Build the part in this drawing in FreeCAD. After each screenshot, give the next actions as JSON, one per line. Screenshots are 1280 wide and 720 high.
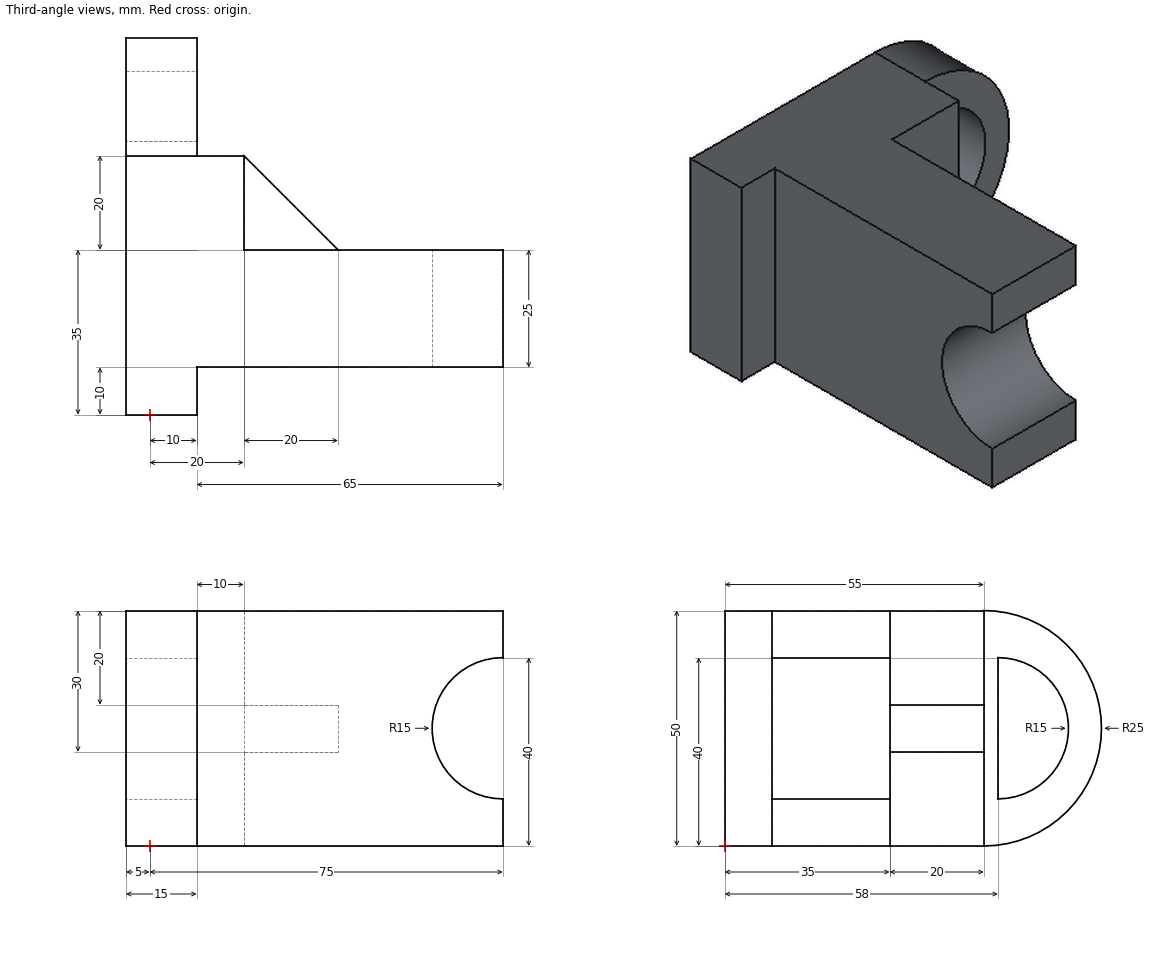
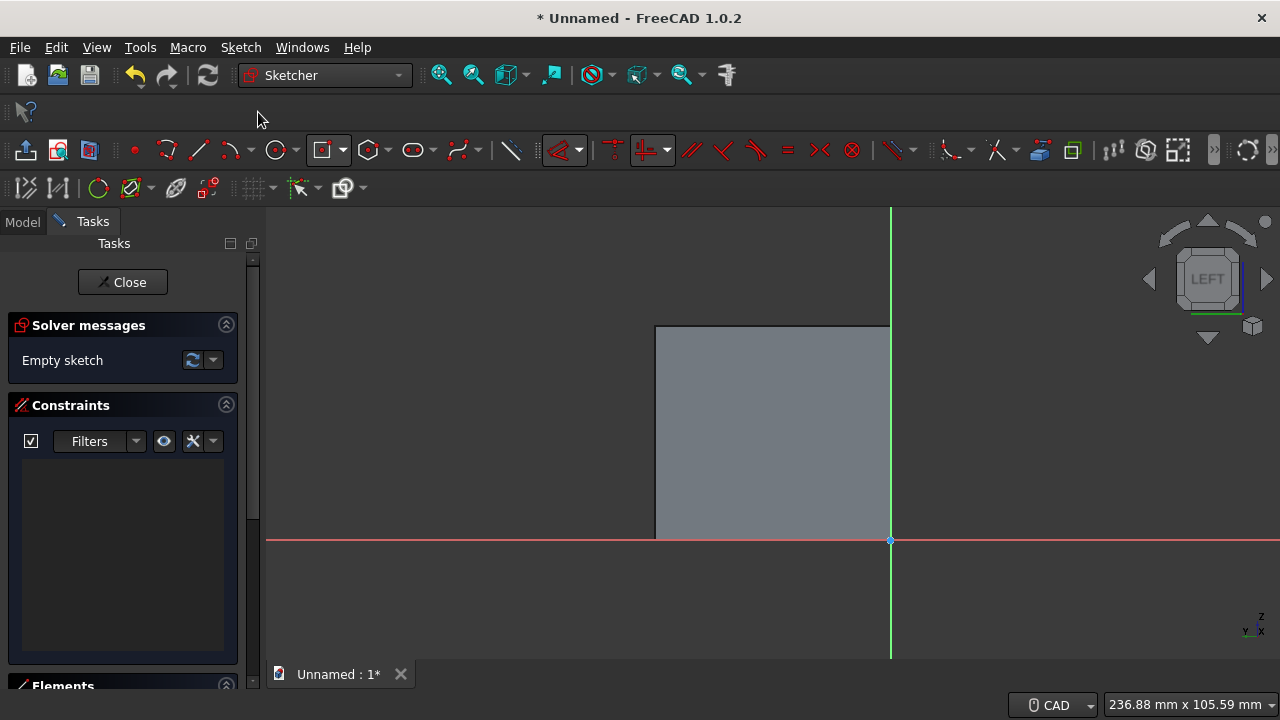
{"action": "left_click", "coordinate": [346, 150]}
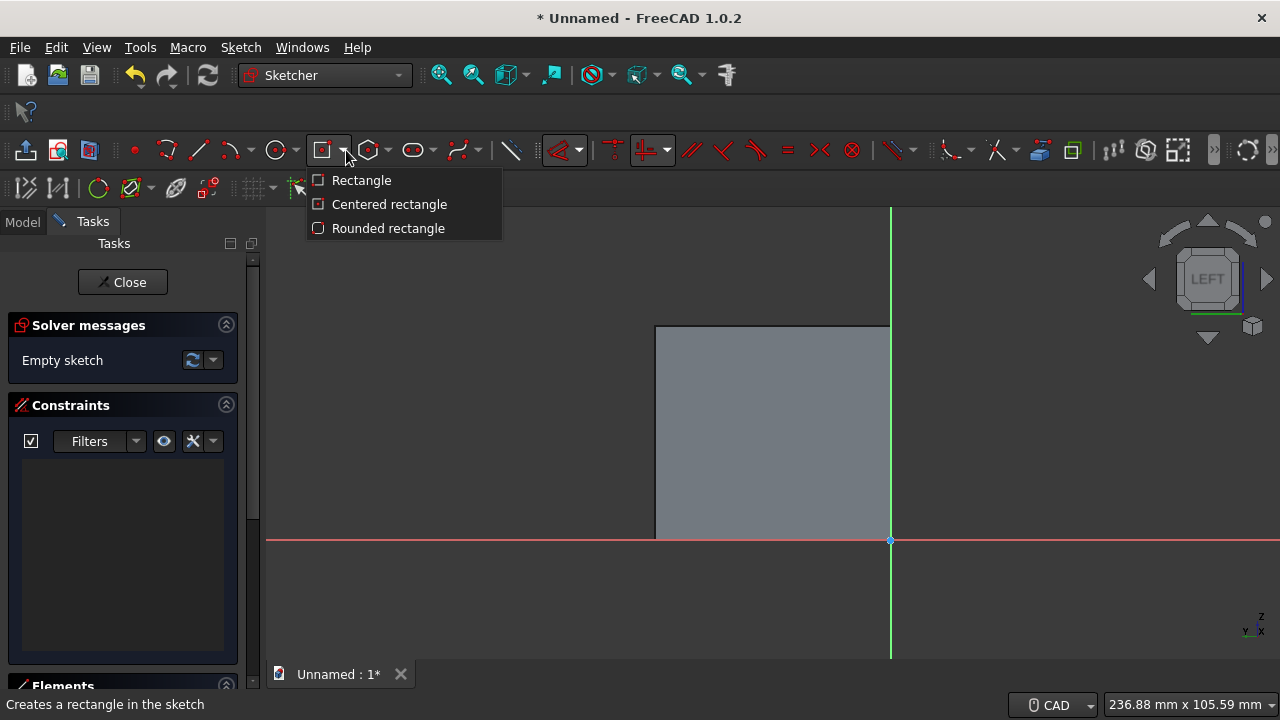
{"action": "left_click", "coordinate": [404, 180]}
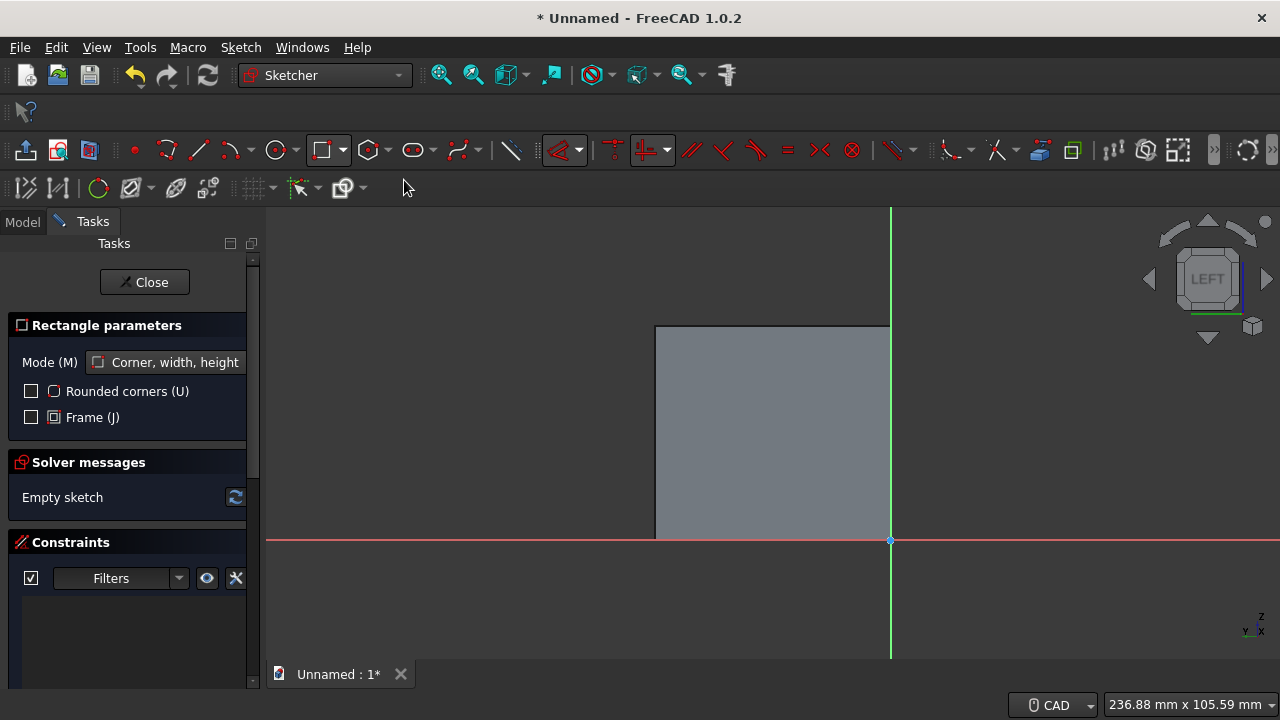
{"action": "left_click", "coordinate": [891, 540]}
{"action": "left_click", "coordinate": [655, 326]}
{"action": "key", "text": "Escape"}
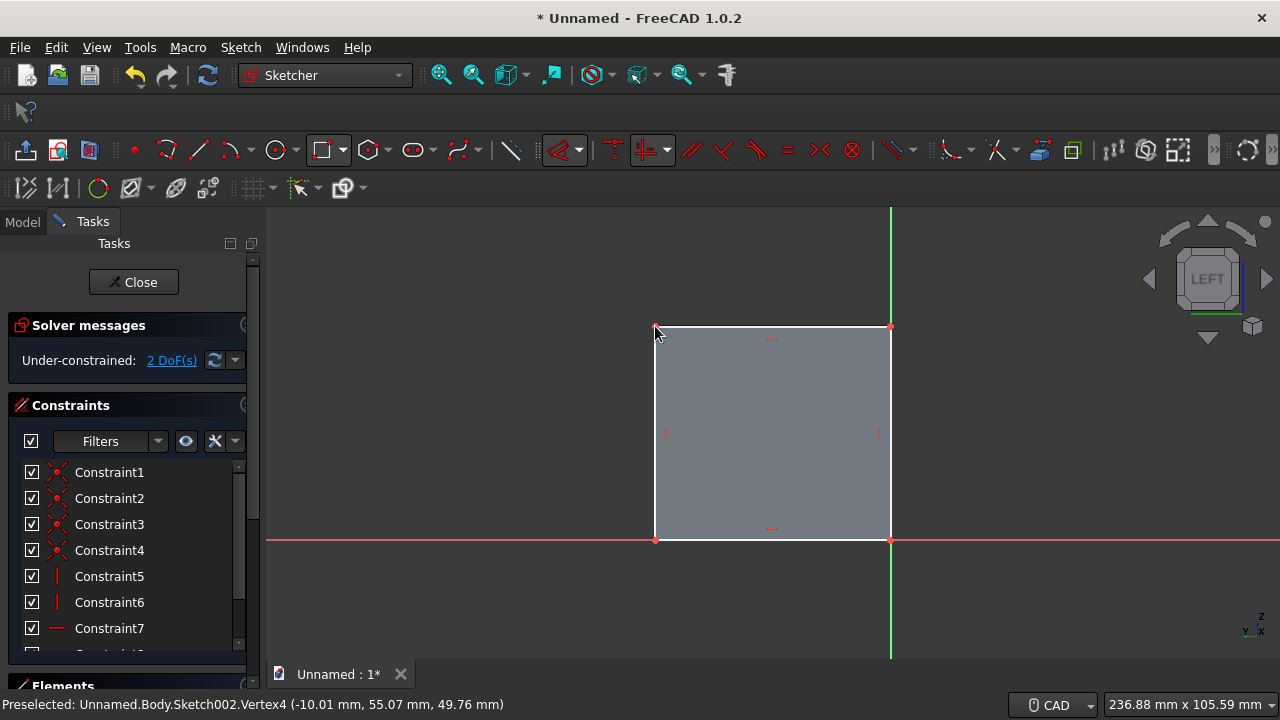
{"action": "left_click", "coordinate": [891, 476]}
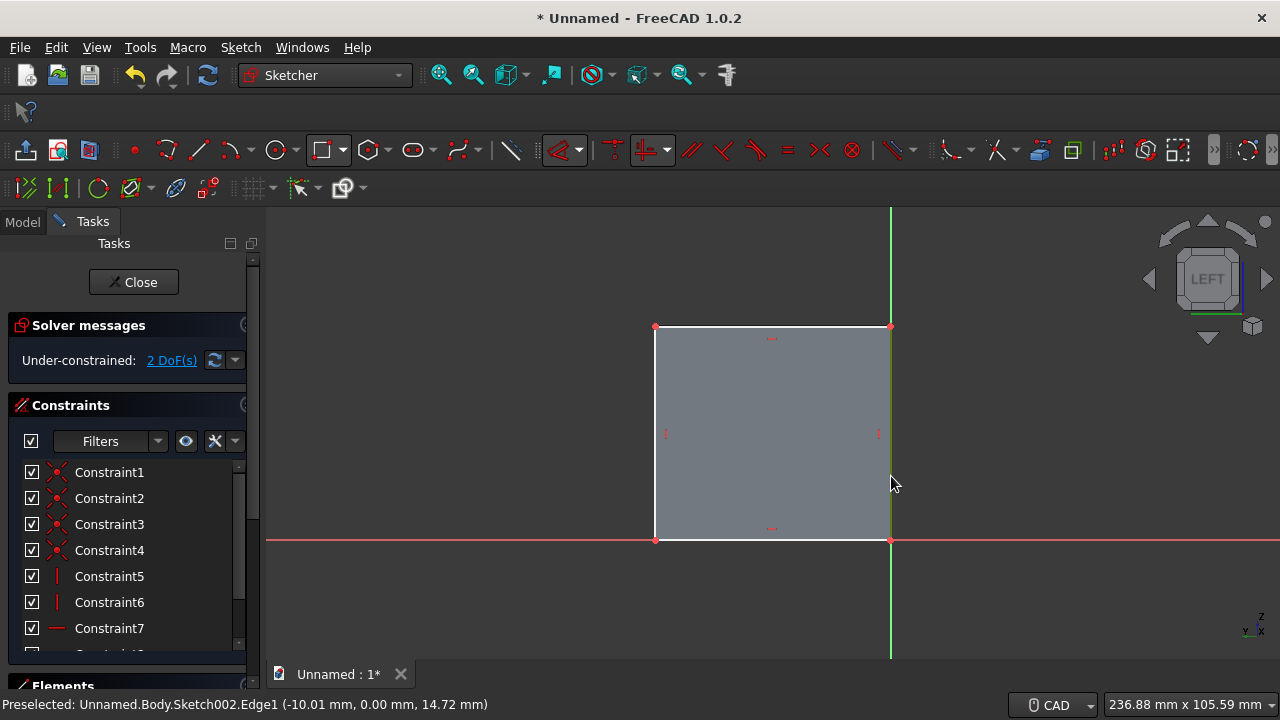
{"action": "left_click", "coordinate": [582, 150]}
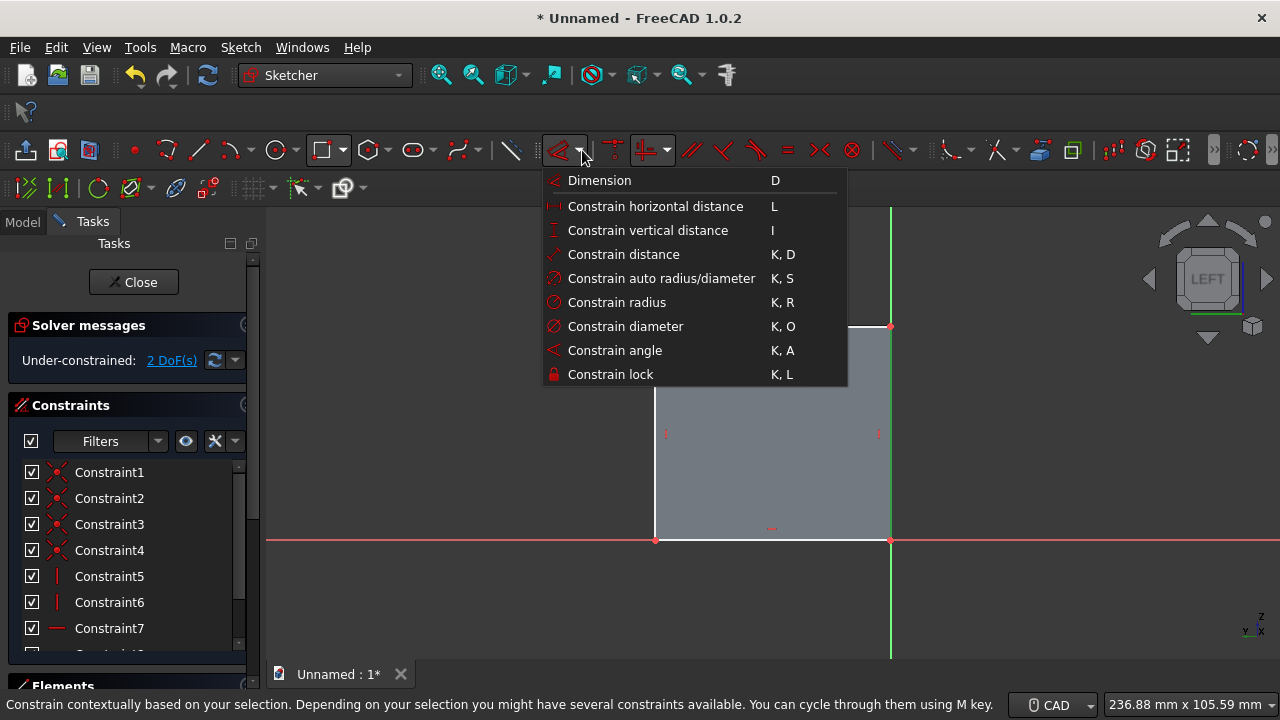
{"action": "left_click", "coordinate": [695, 230]}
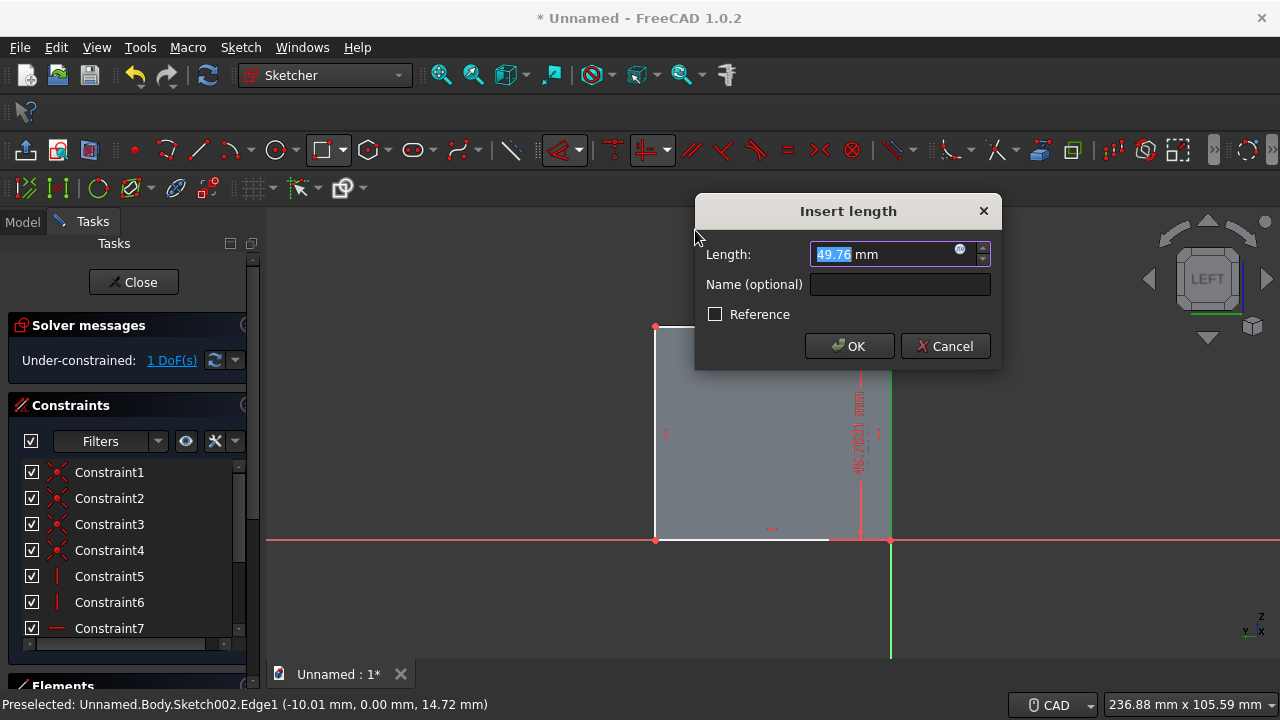
{"action": "type", "text": "50"}
{"action": "key", "text": "Return"}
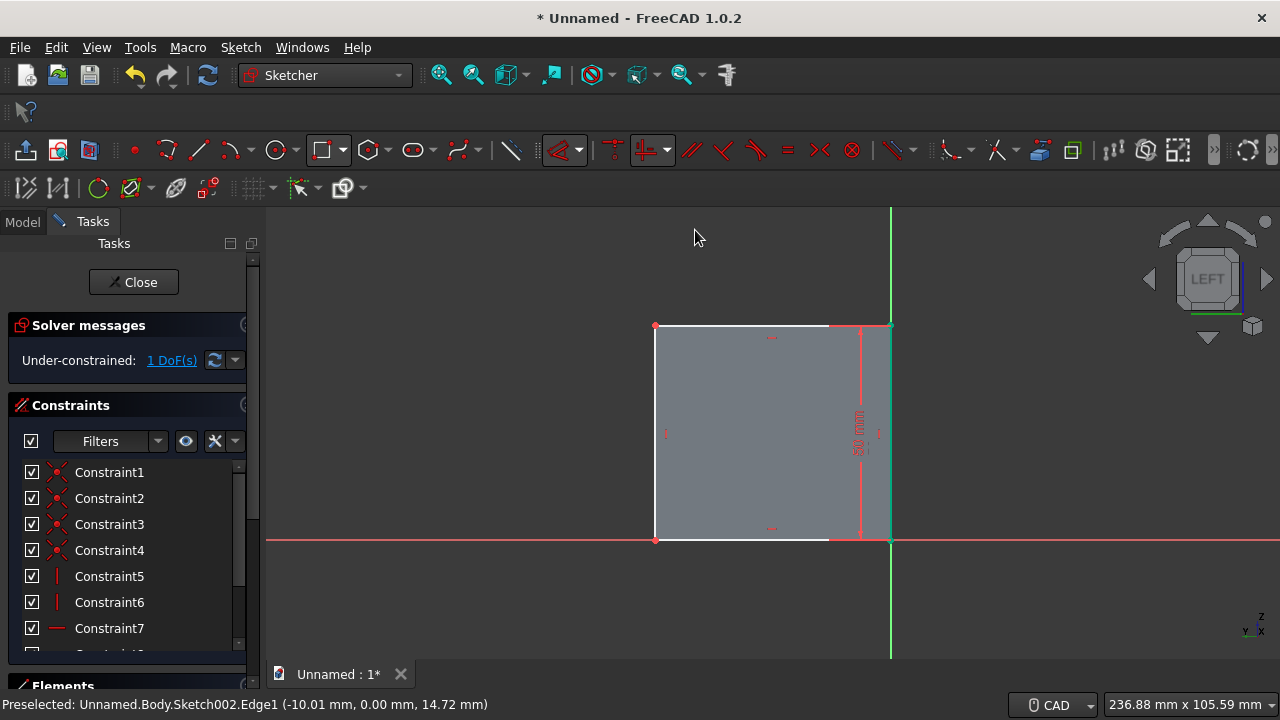
{"action": "left_click", "coordinate": [820, 326]}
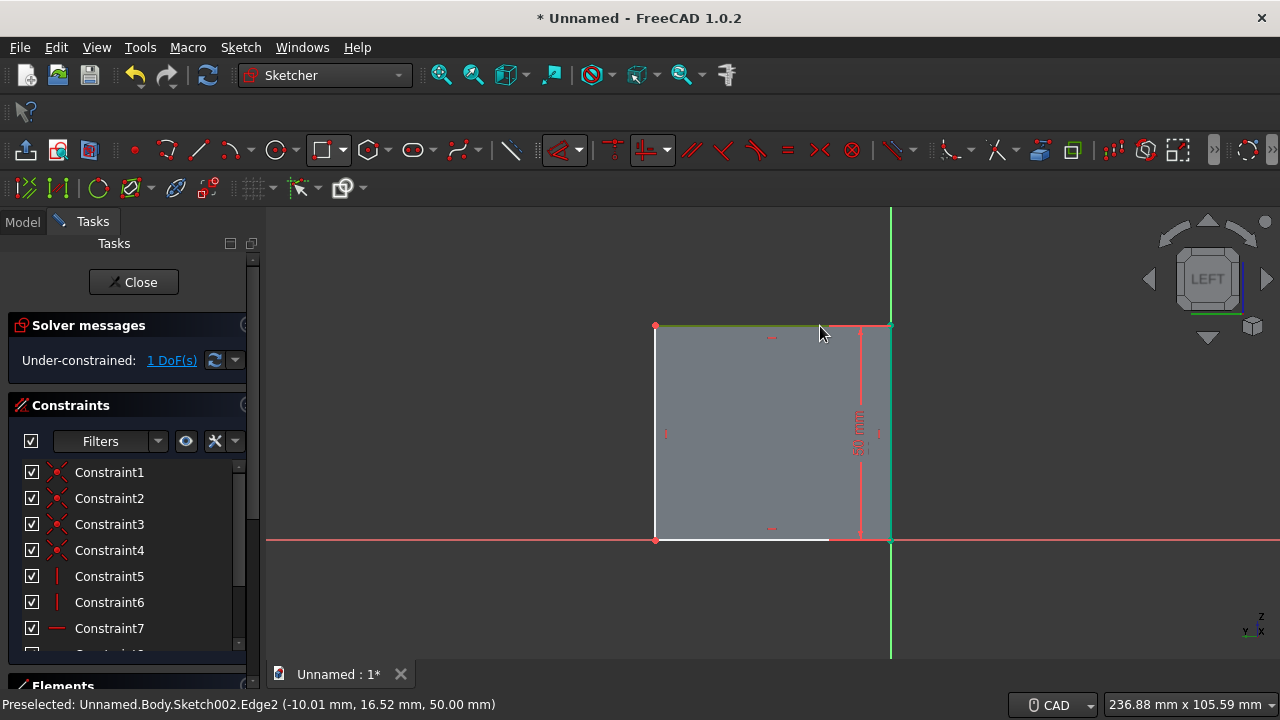
{"action": "left_click", "coordinate": [582, 150]}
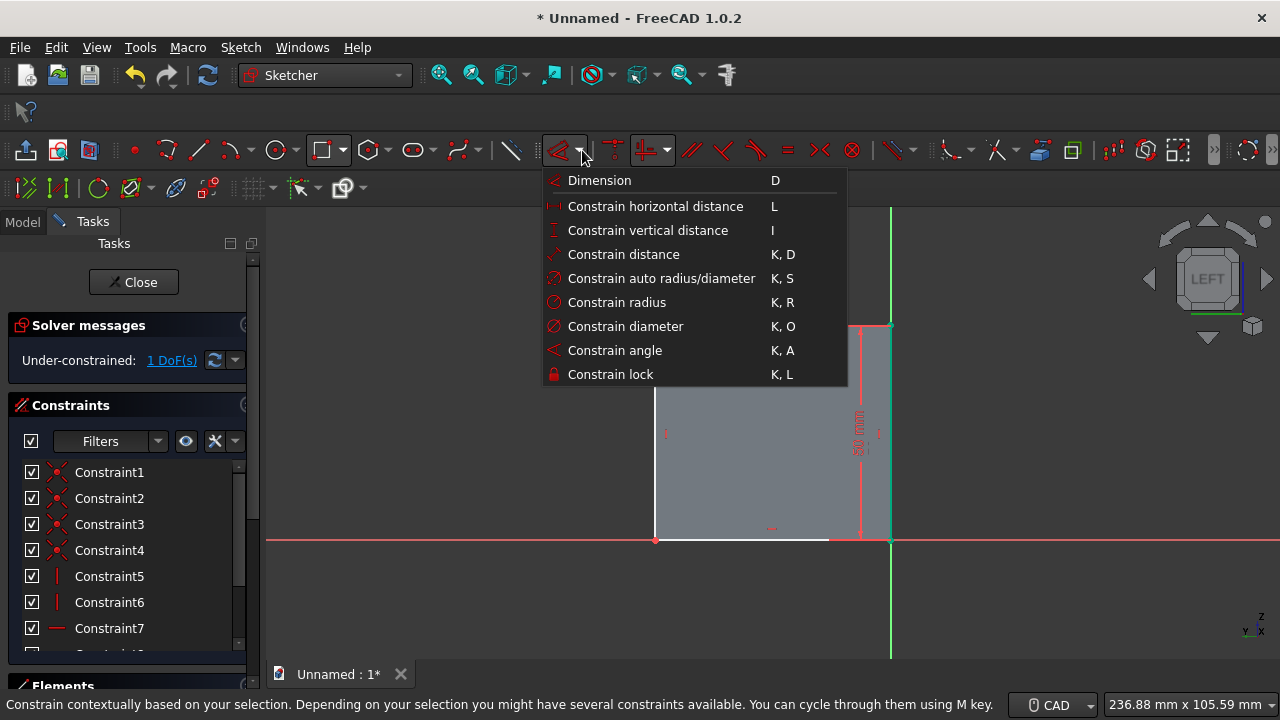
{"action": "left_click", "coordinate": [695, 206]}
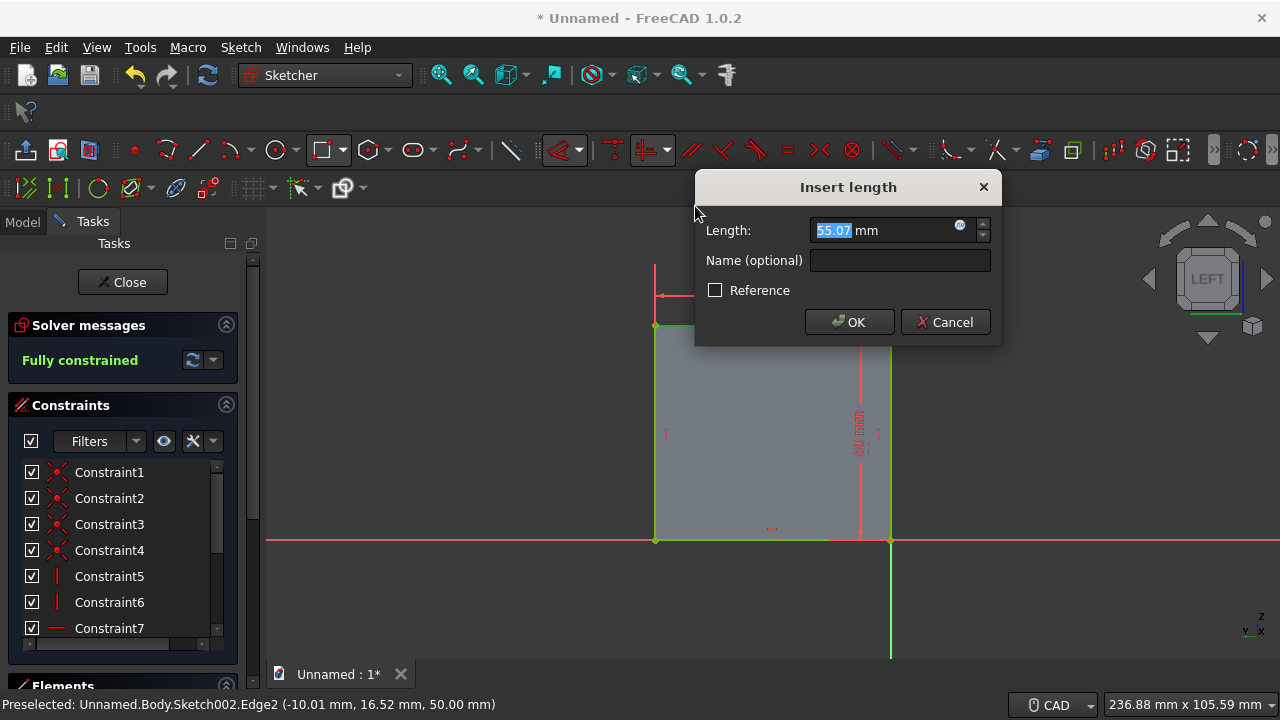
{"action": "type", "text": "55"}
{"action": "key", "text": "Return"}